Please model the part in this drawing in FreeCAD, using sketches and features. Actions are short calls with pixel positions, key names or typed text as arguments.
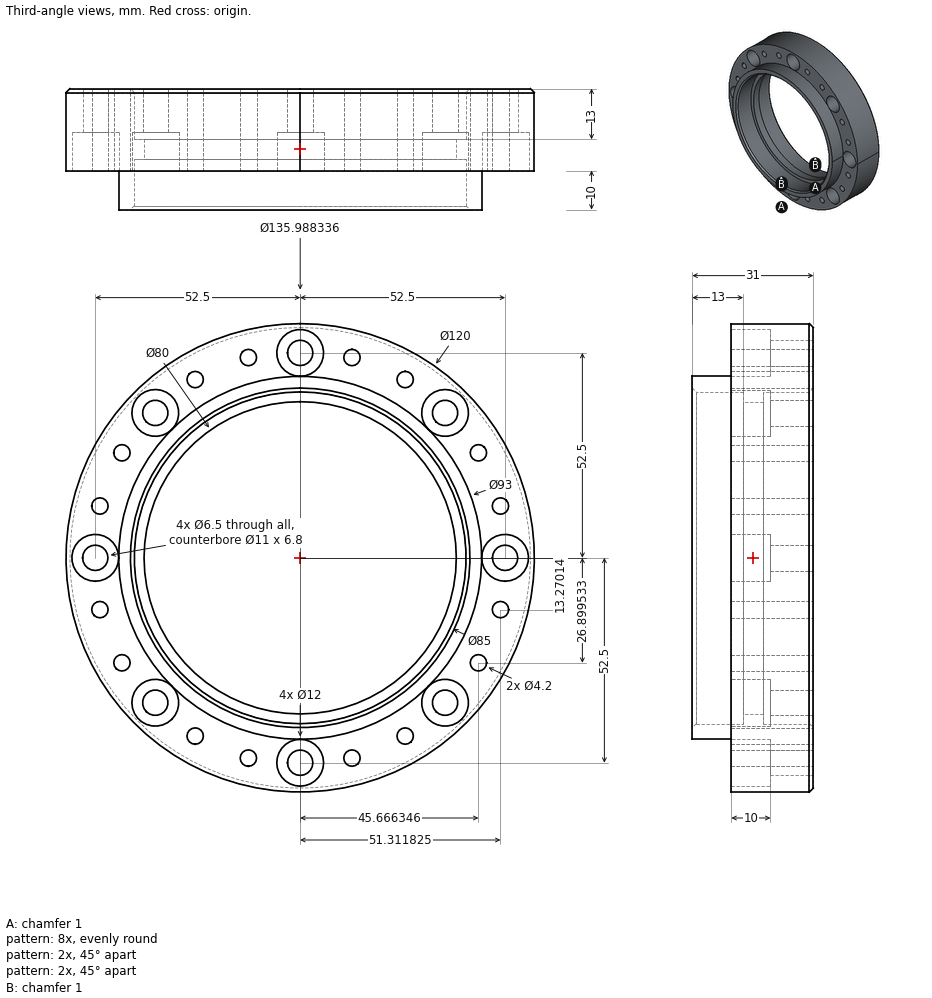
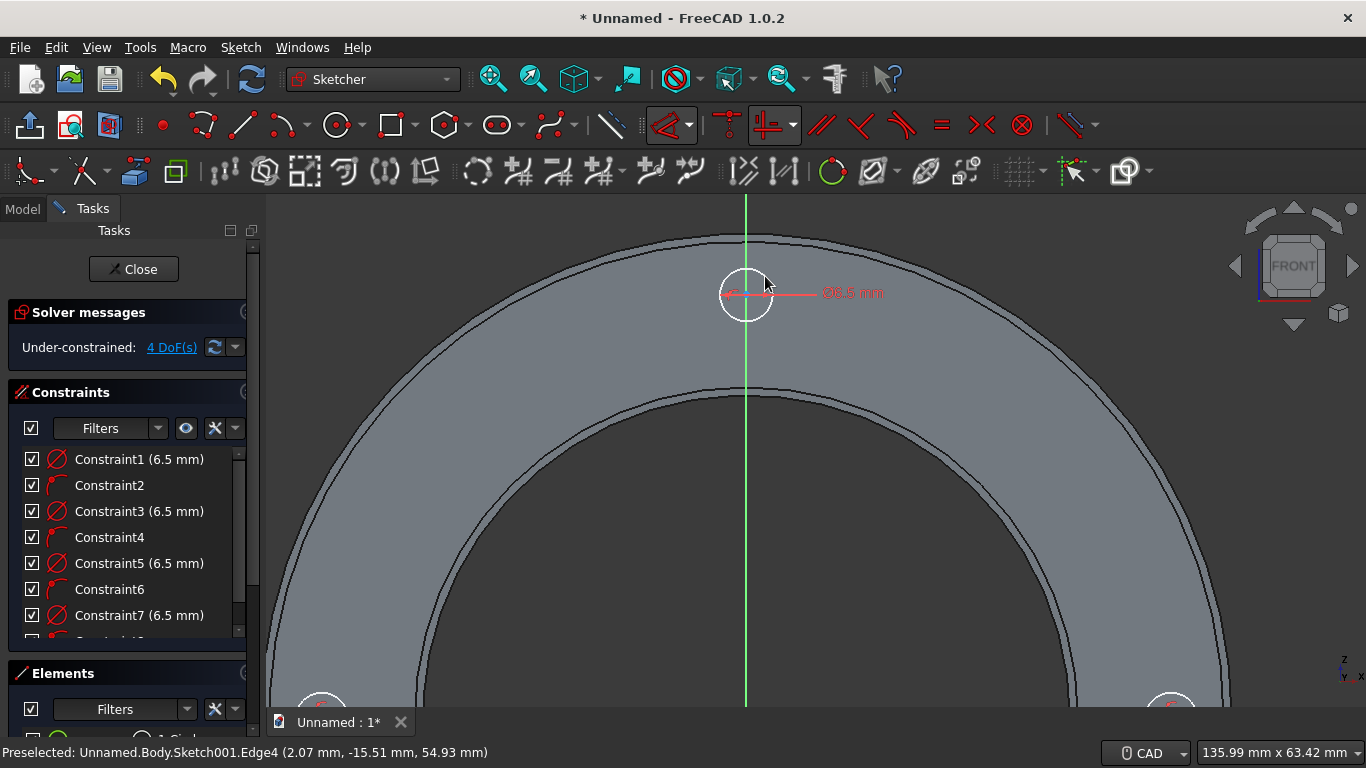
click(666, 126)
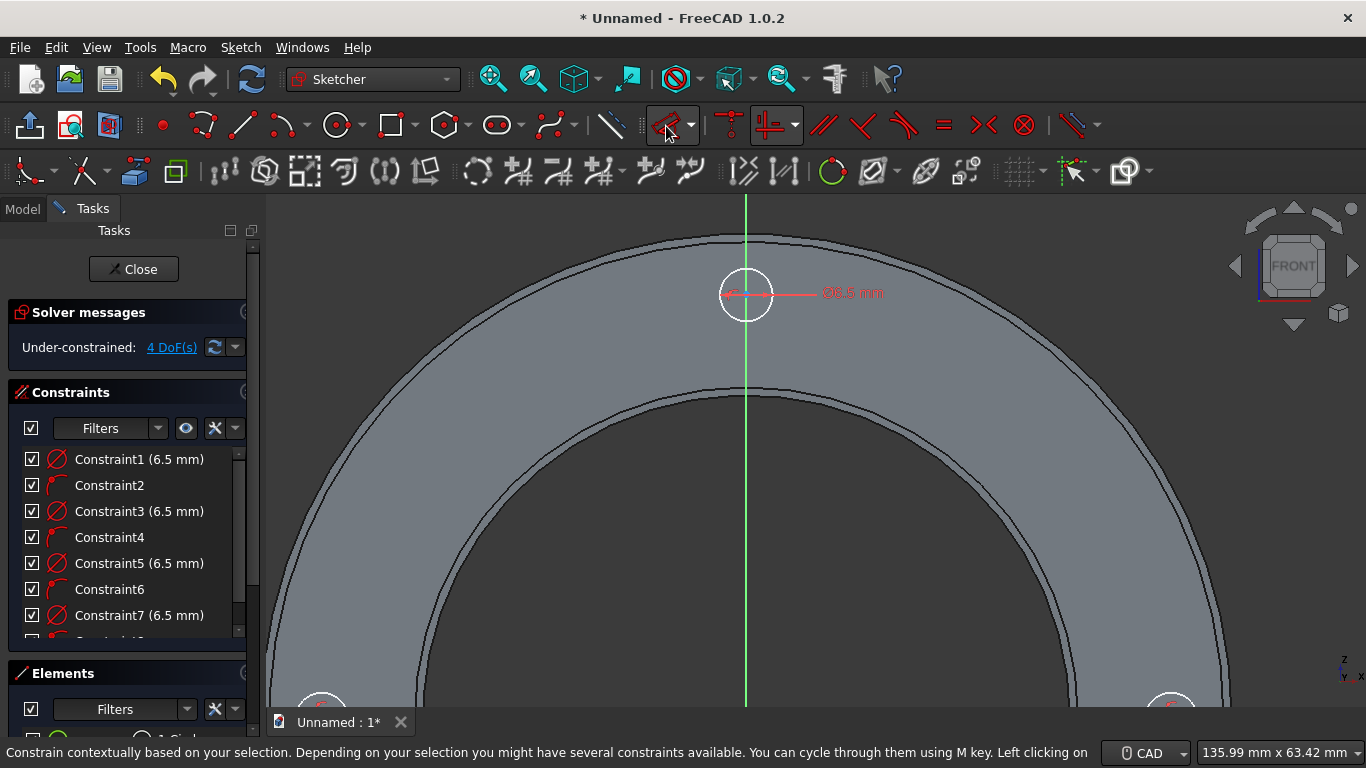
scroll(748, 294, down, 5)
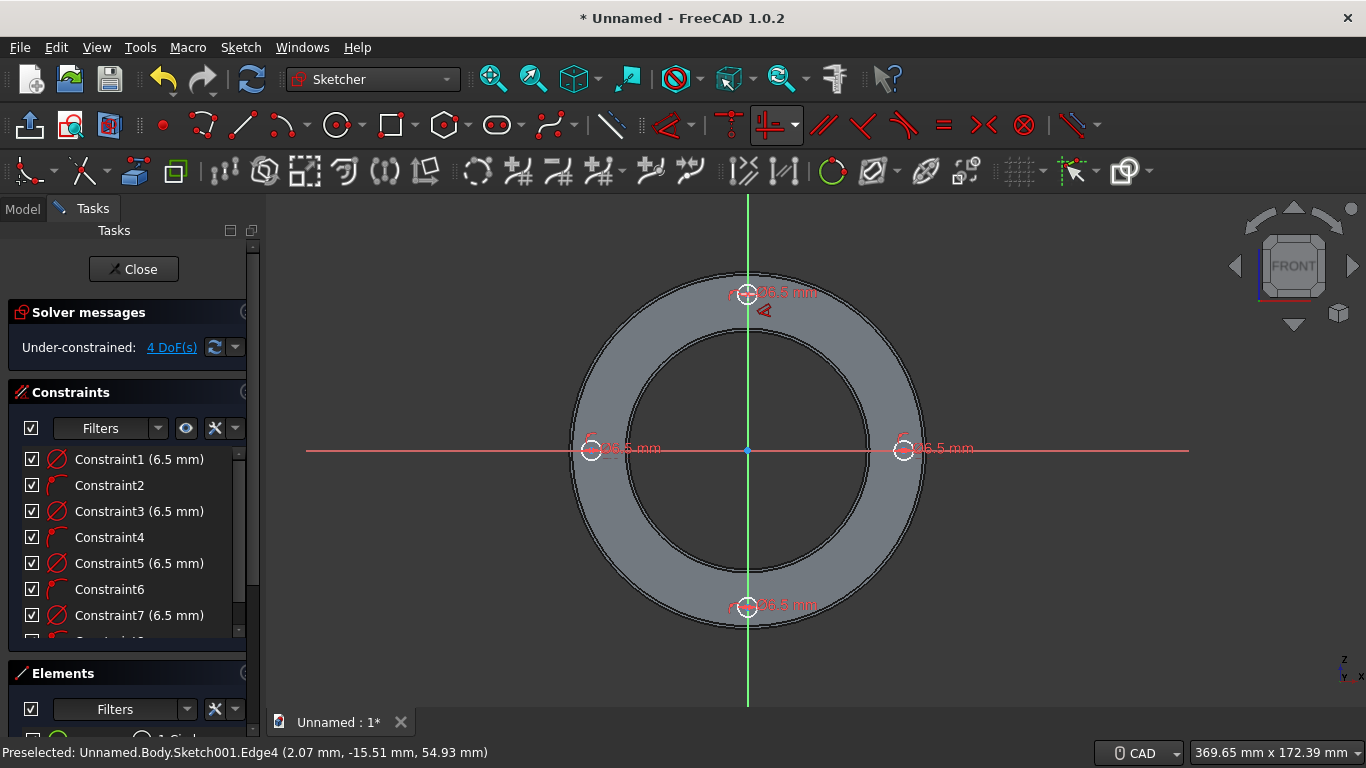
click(592, 451)
click(670, 485)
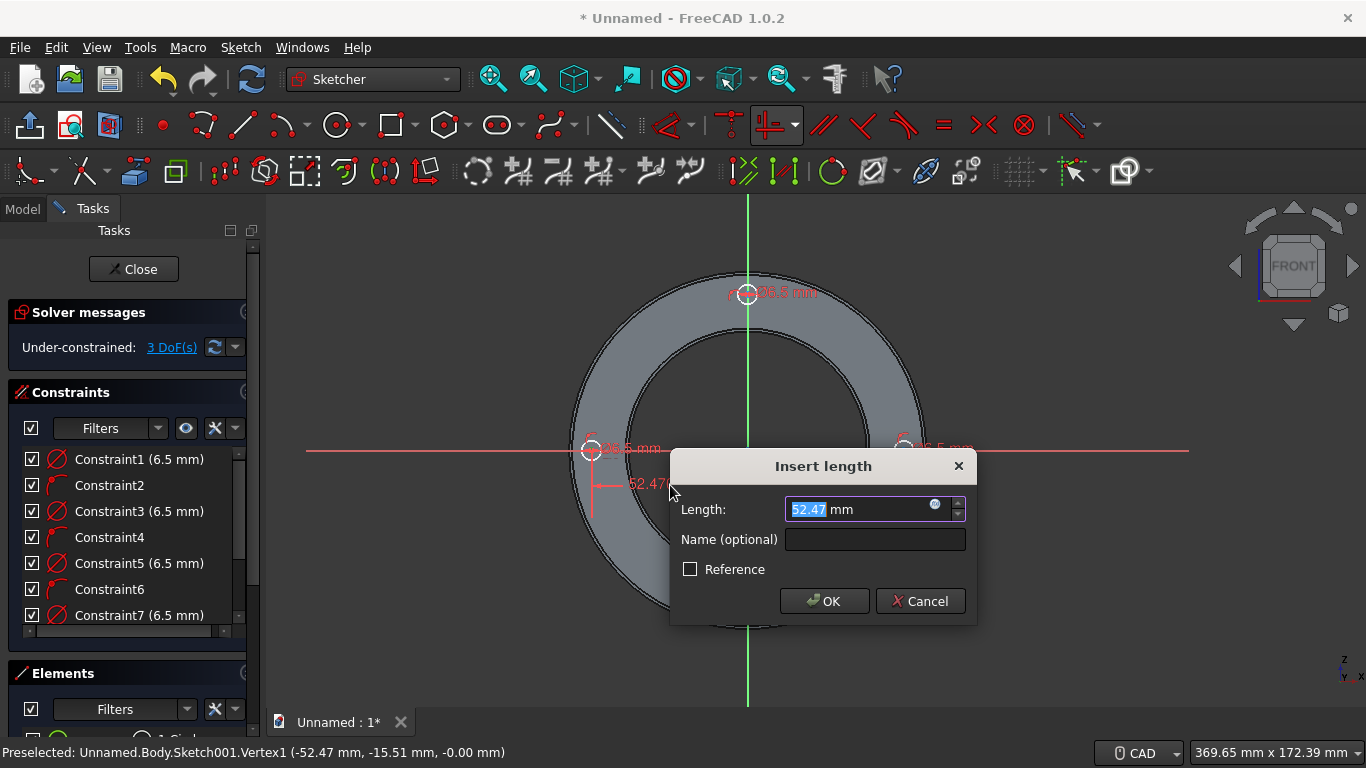
text(52.5)
key(Return)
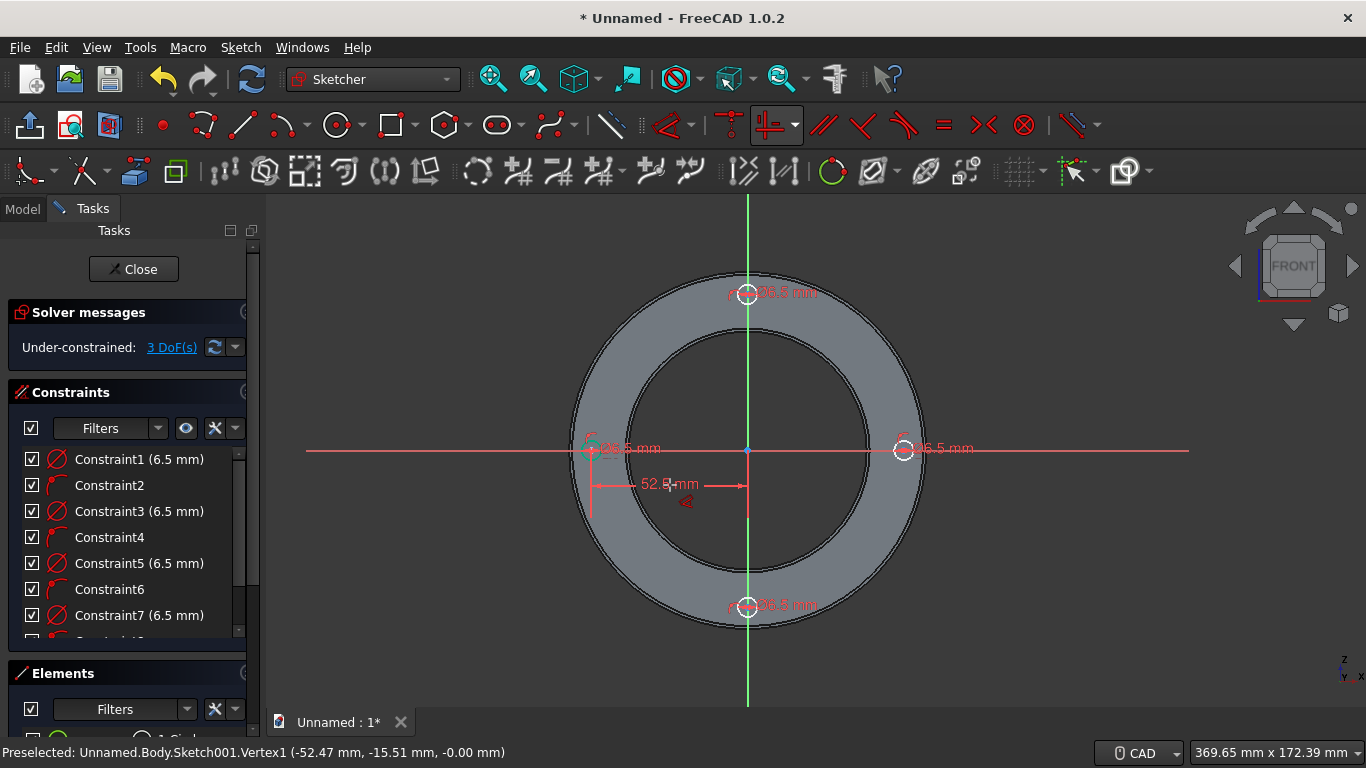
click(904, 451)
click(826, 485)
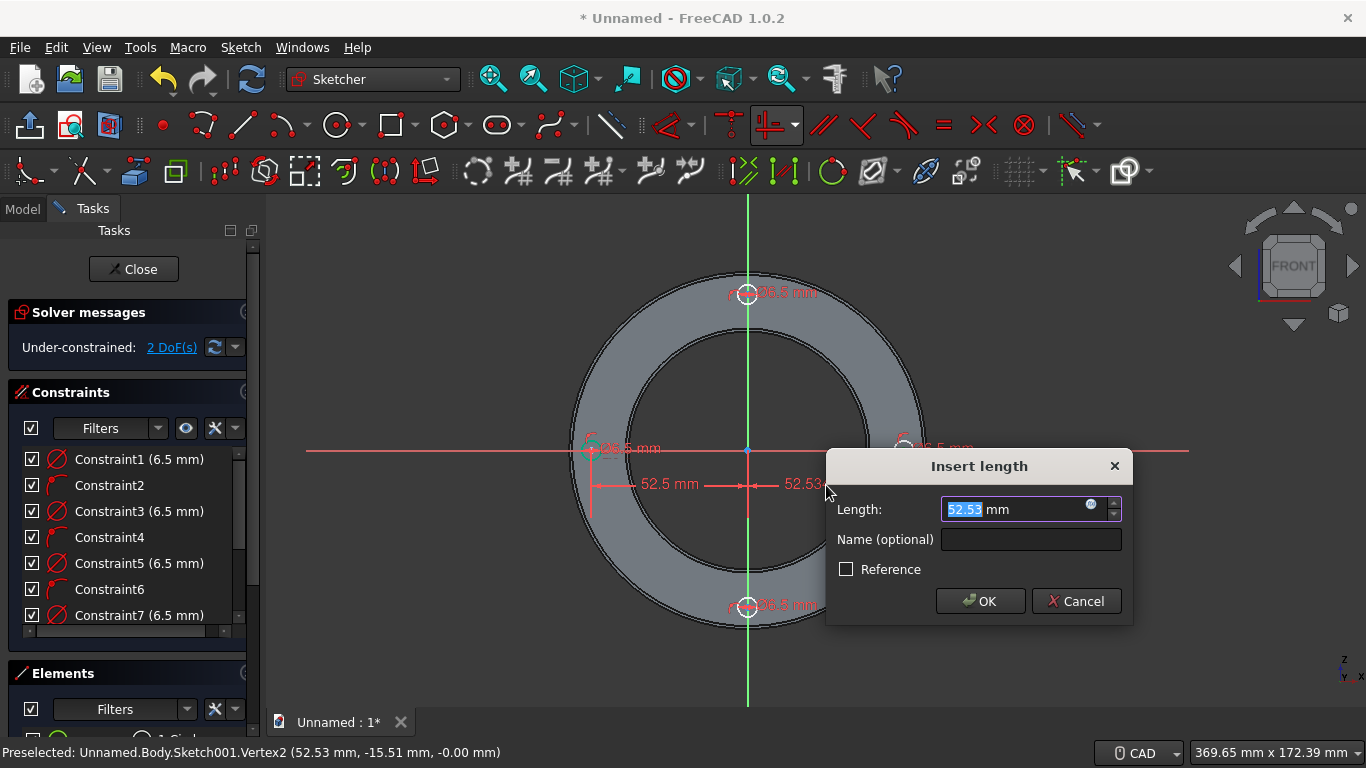
text(52.5)
key(Return)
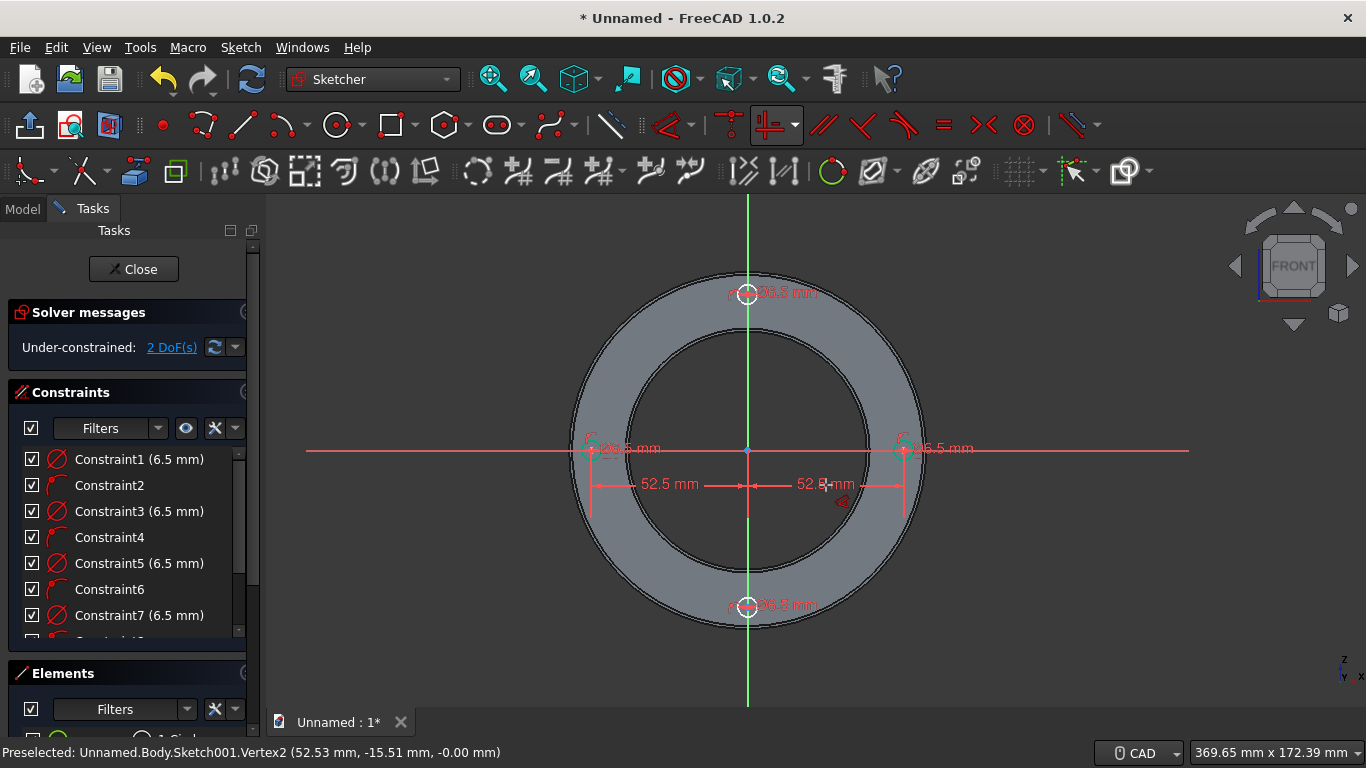
click(748, 607)
click(782, 529)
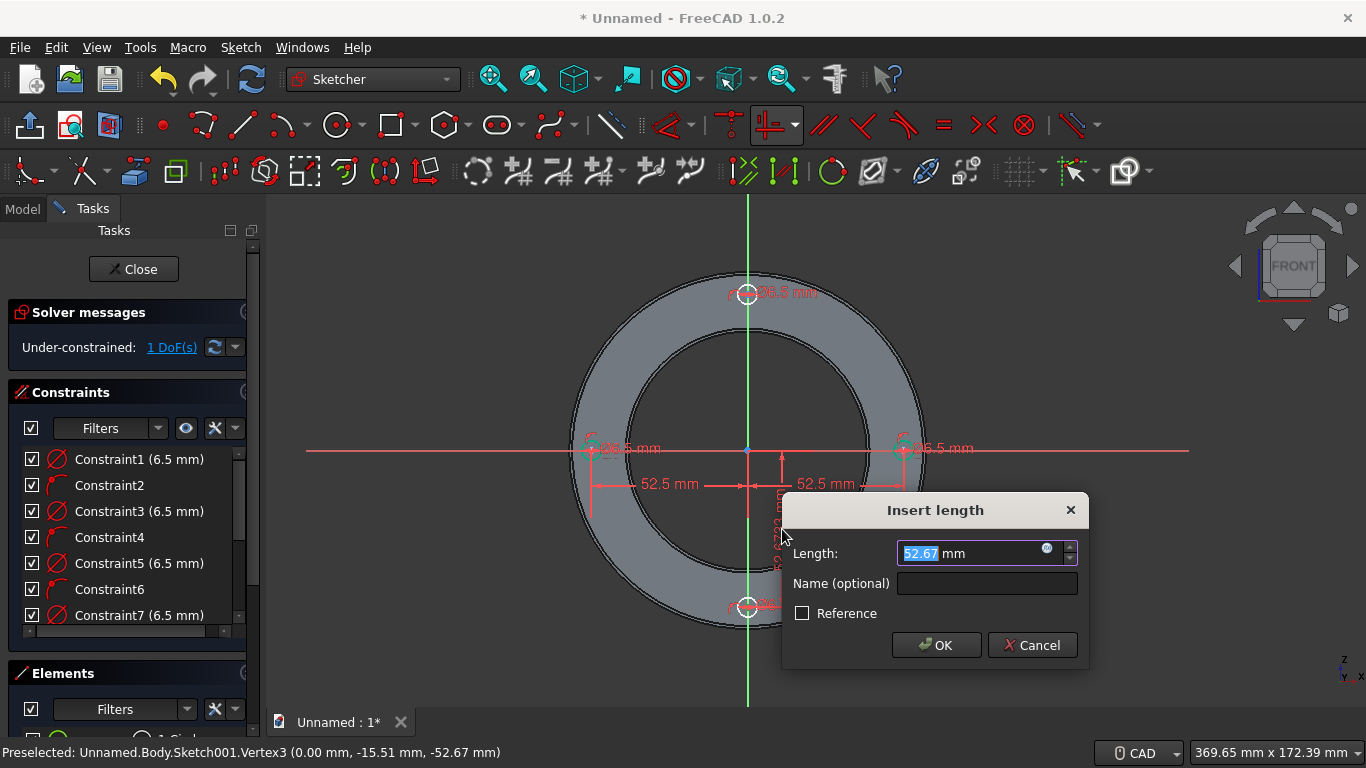
text(52.5)
key(Return)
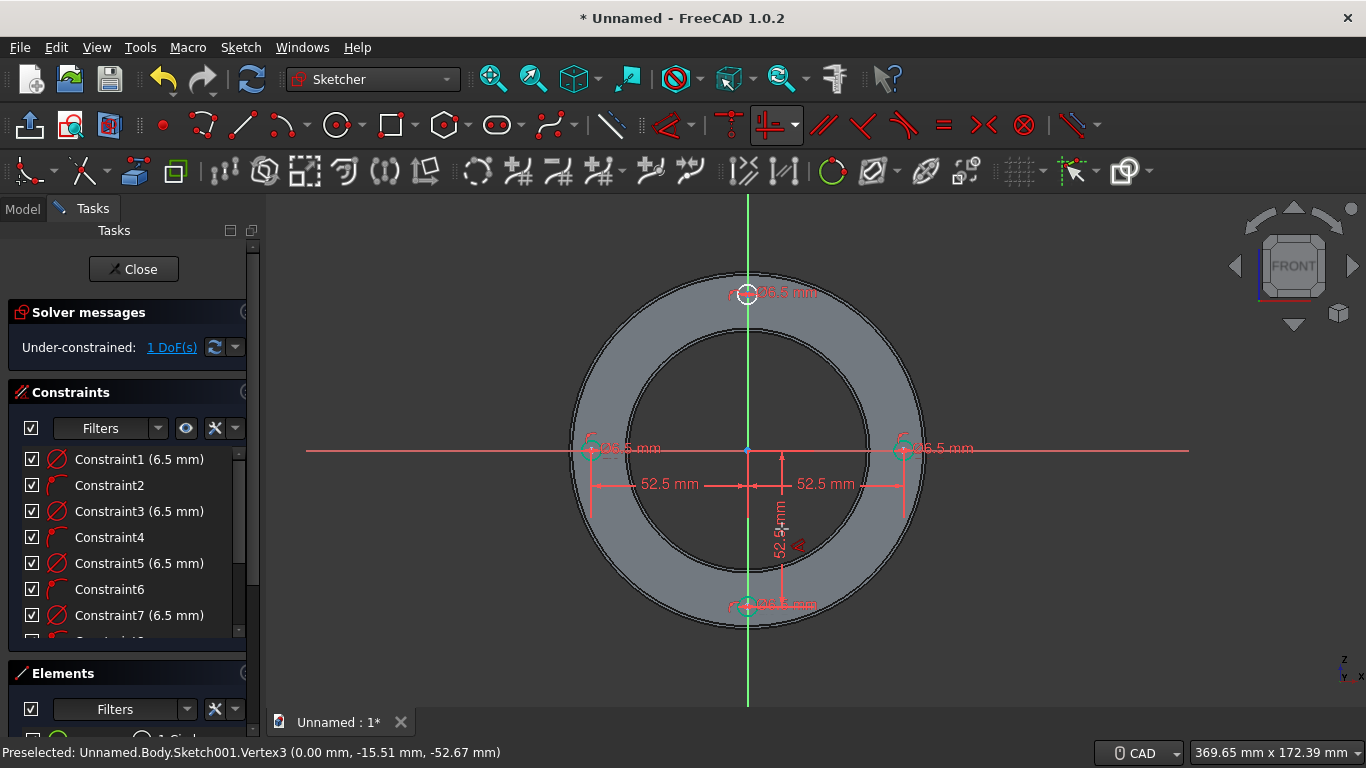
click(748, 294)
click(782, 372)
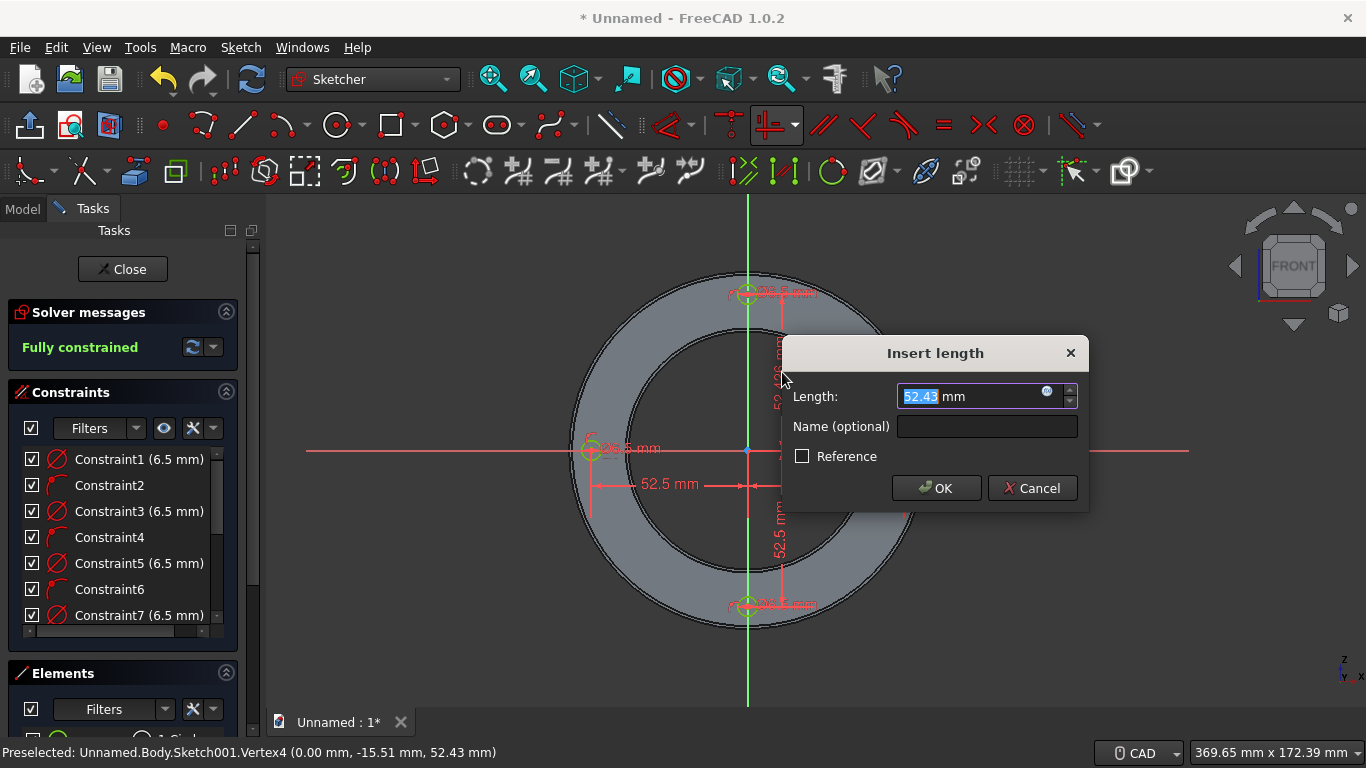
text(52.5)
key(Return)
key(Escape)